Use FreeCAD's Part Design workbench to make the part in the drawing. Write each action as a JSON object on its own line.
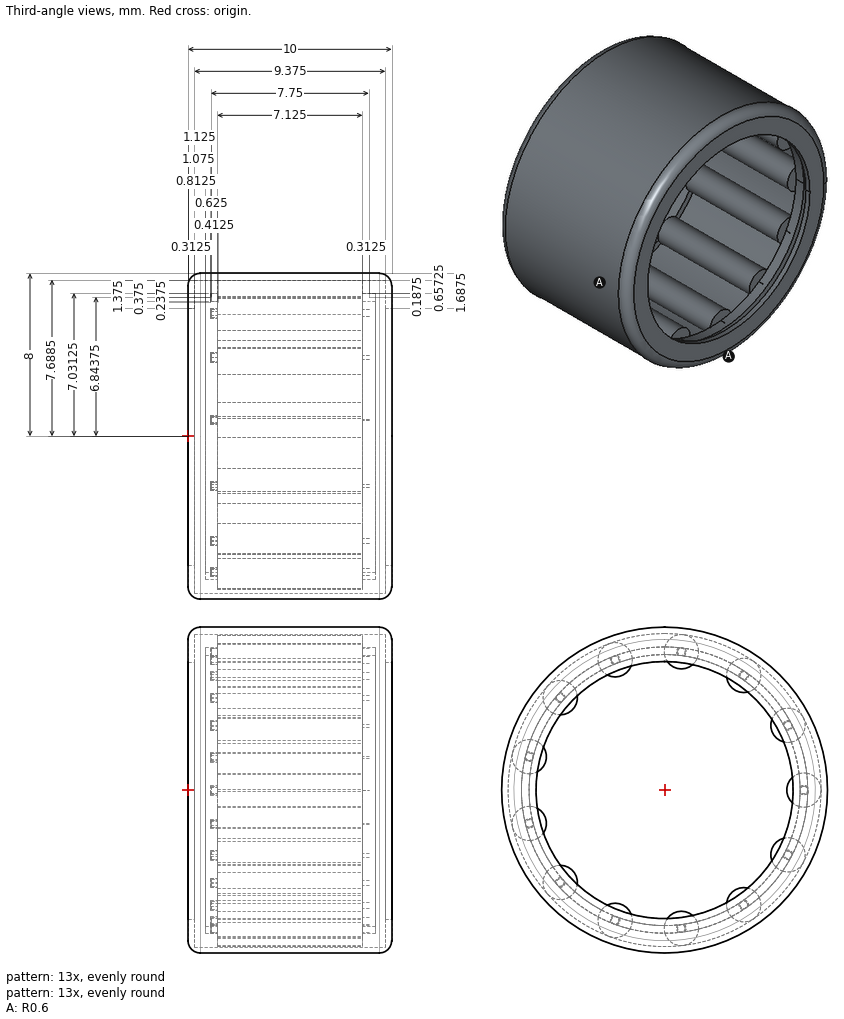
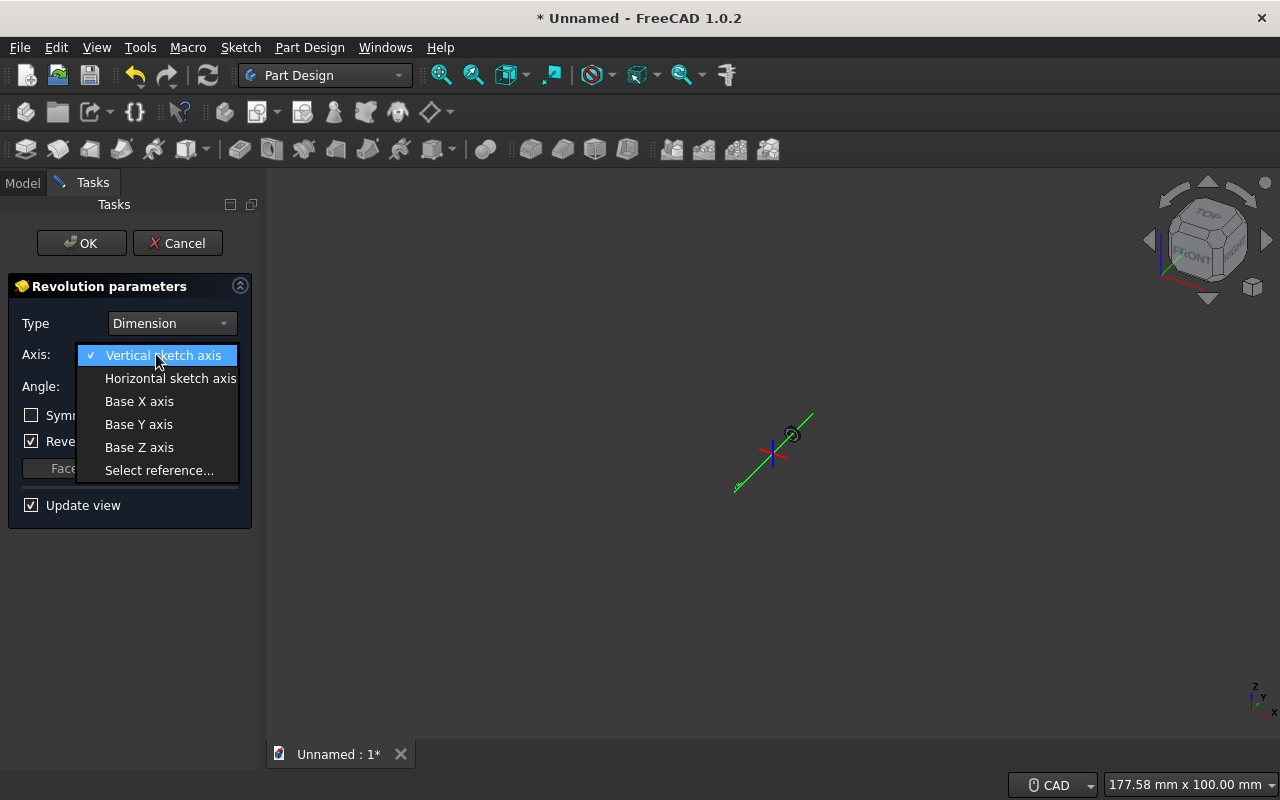
{"action": "left_click", "coordinate": [156, 378]}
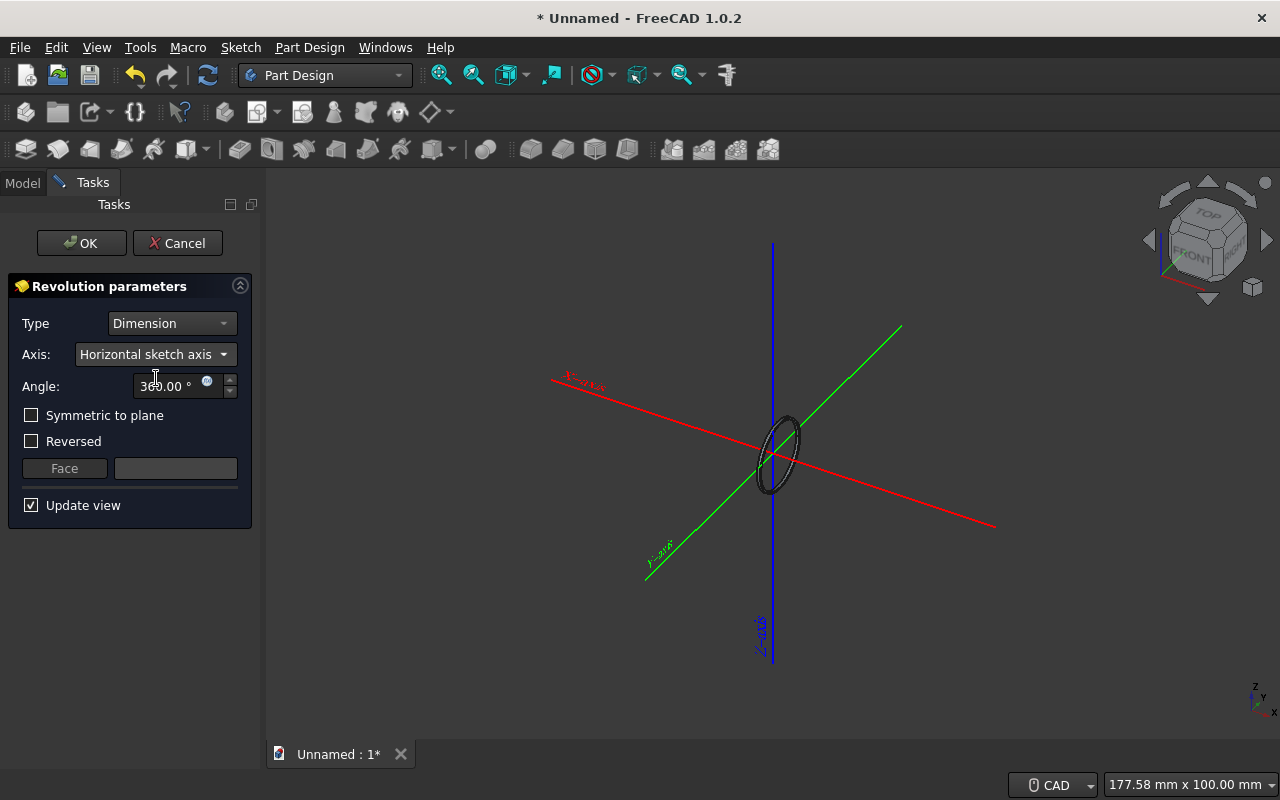
{"action": "left_click", "coordinate": [82, 243]}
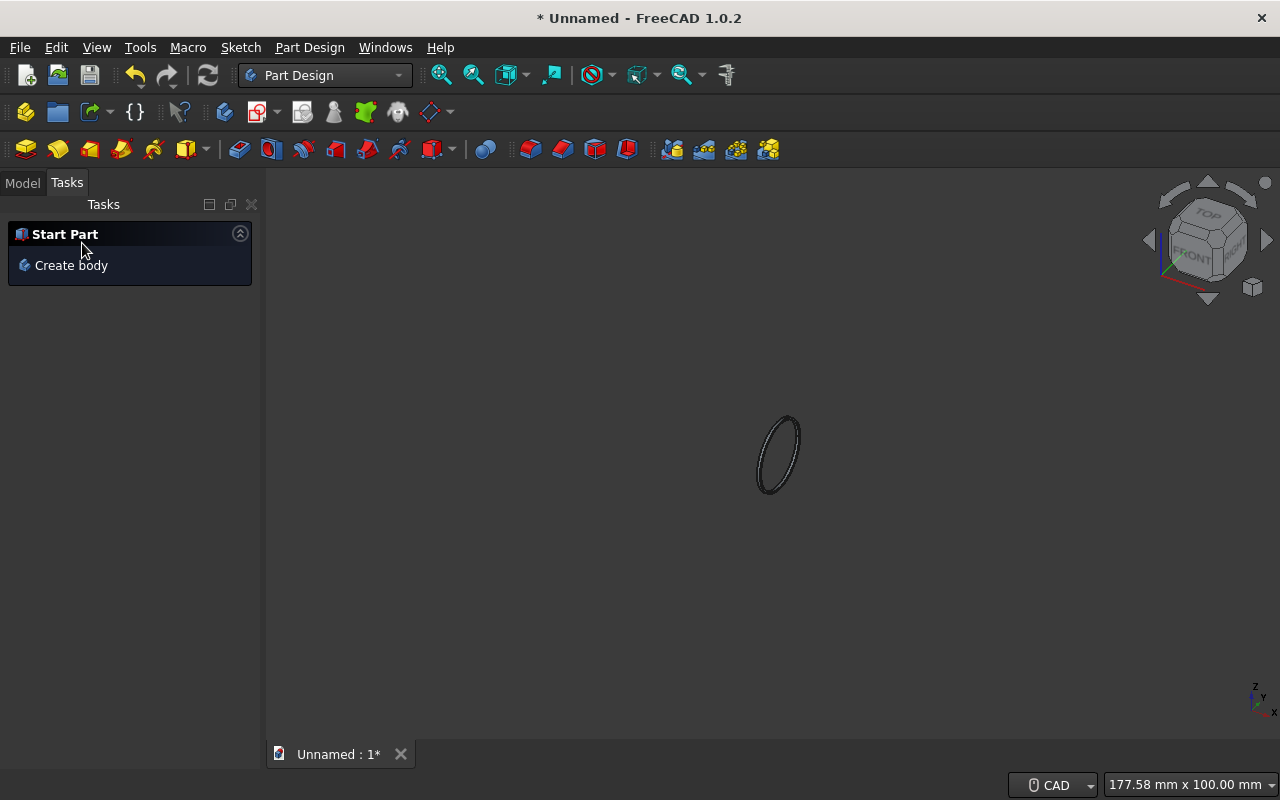
{"action": "left_click", "coordinate": [442, 76]}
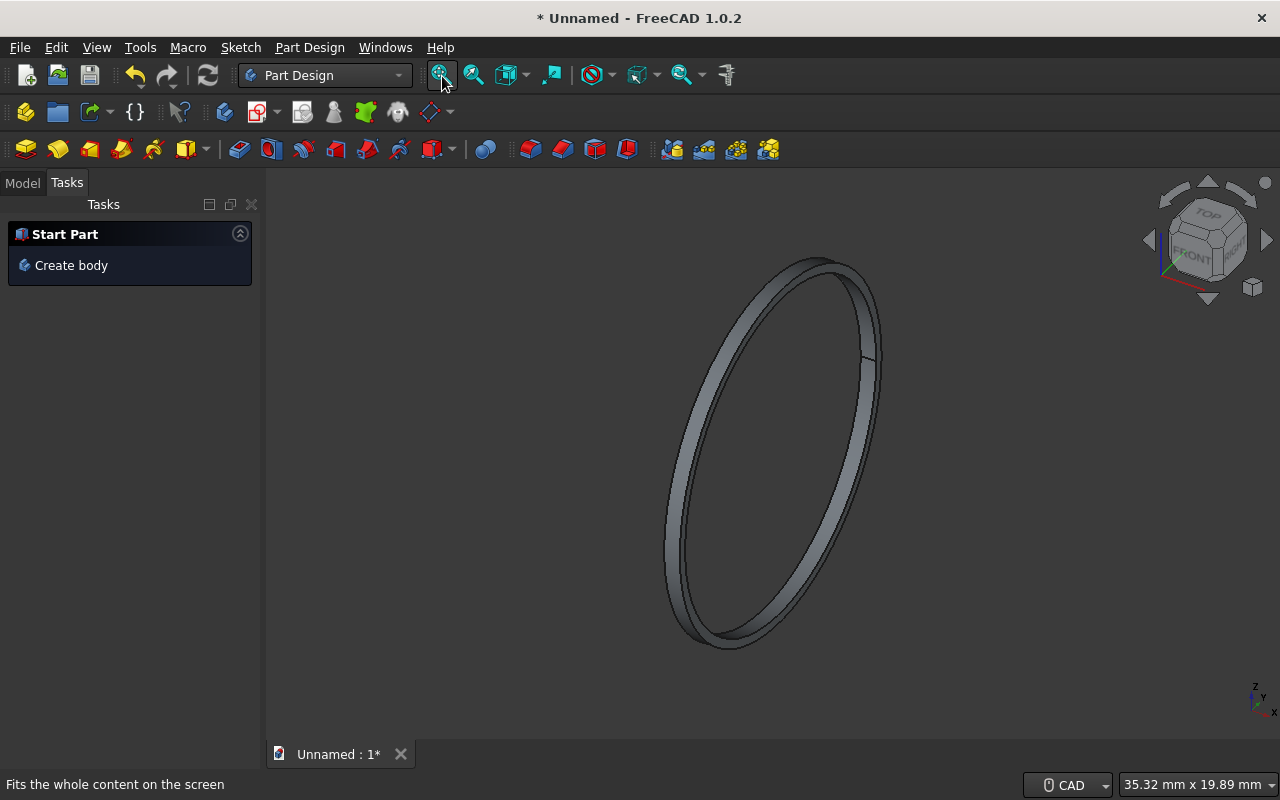
{"action": "left_click", "coordinate": [258, 112]}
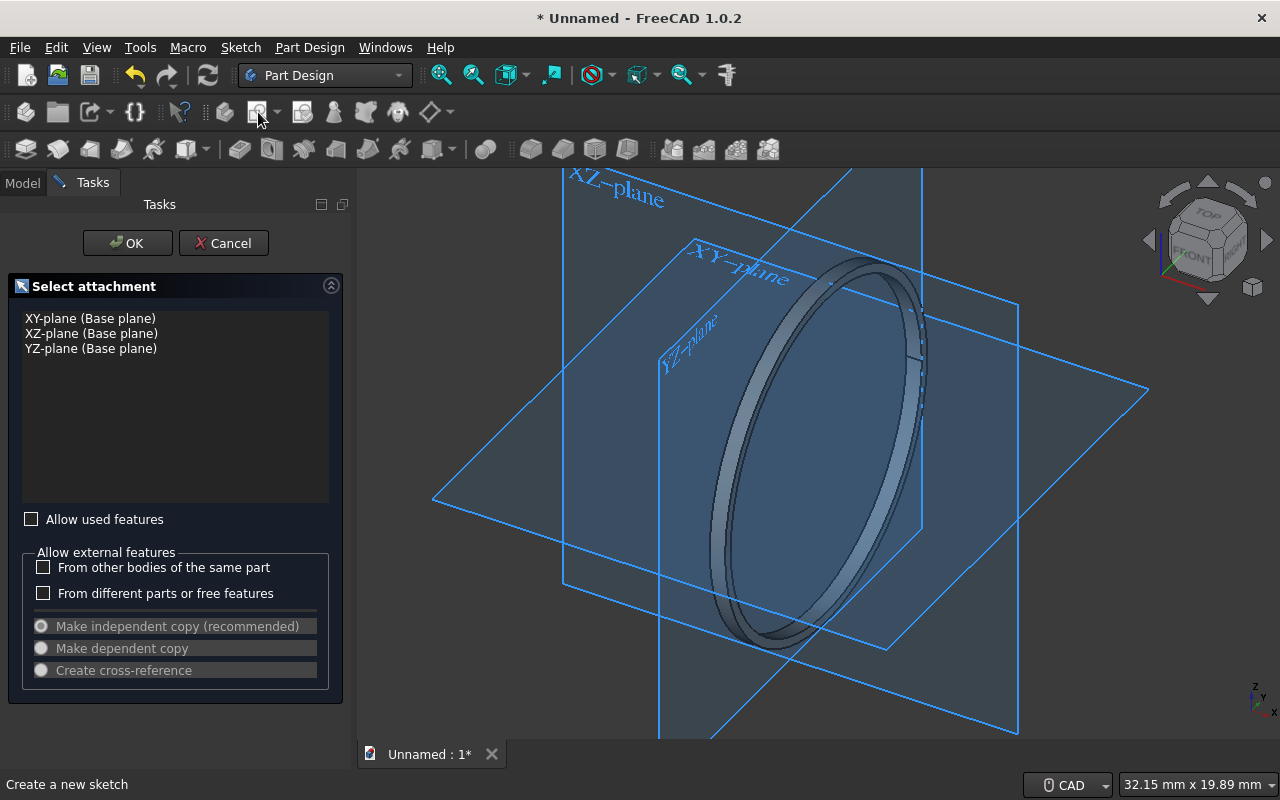
{"action": "left_click", "coordinate": [82, 318]}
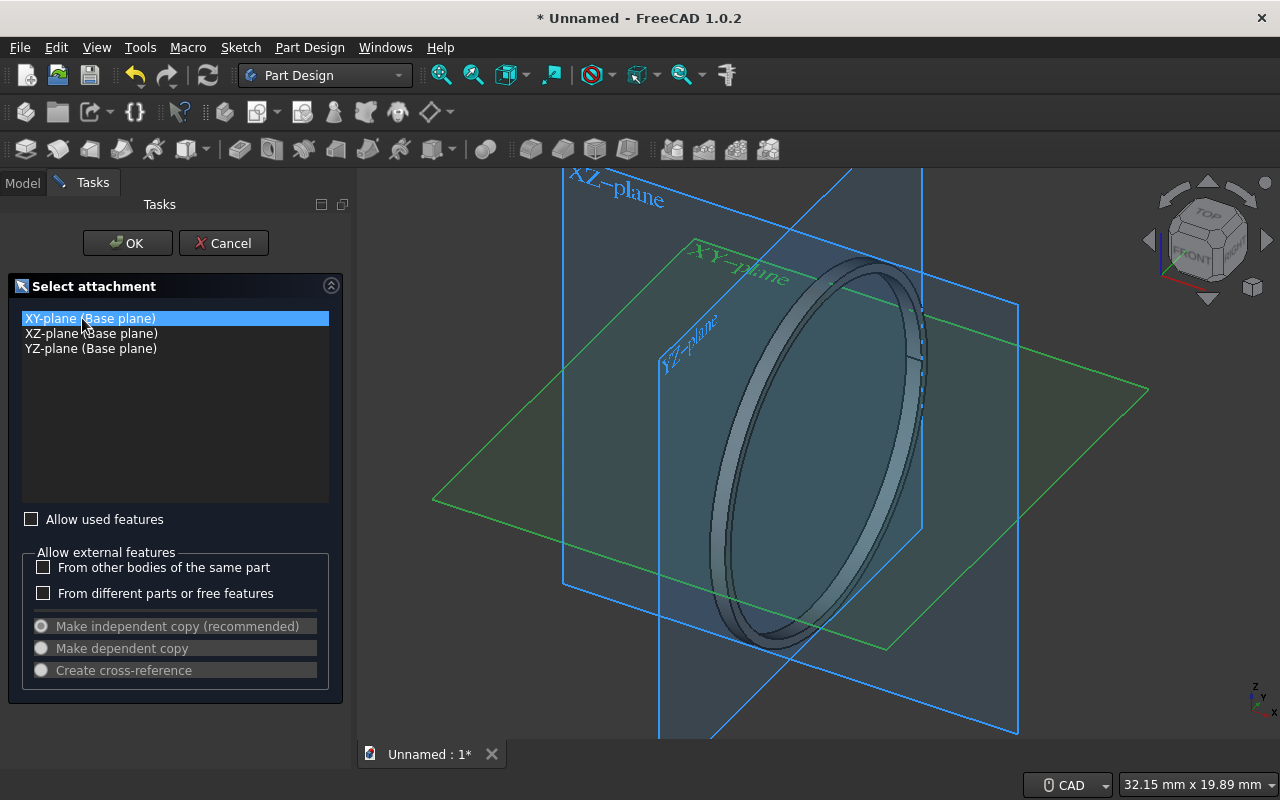
{"action": "left_click", "coordinate": [128, 243]}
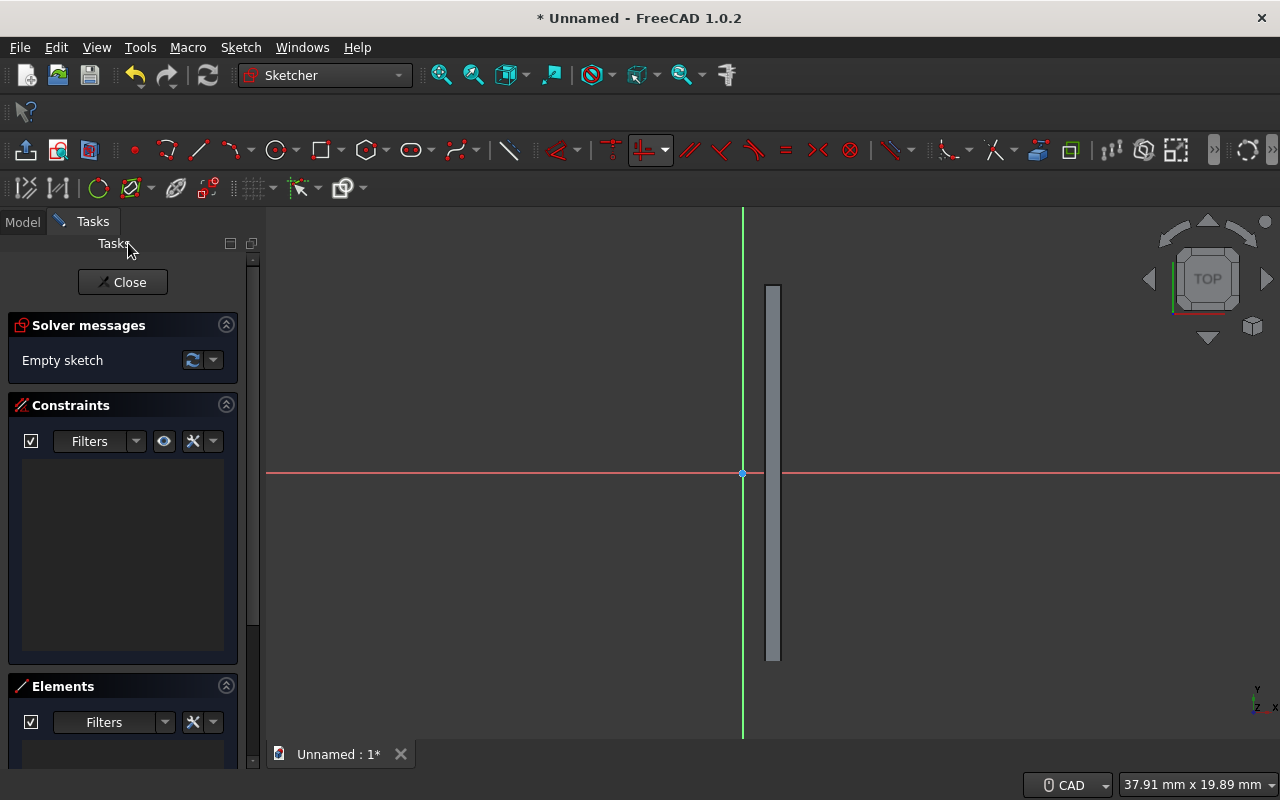
{"action": "left_click", "coordinate": [90, 150]}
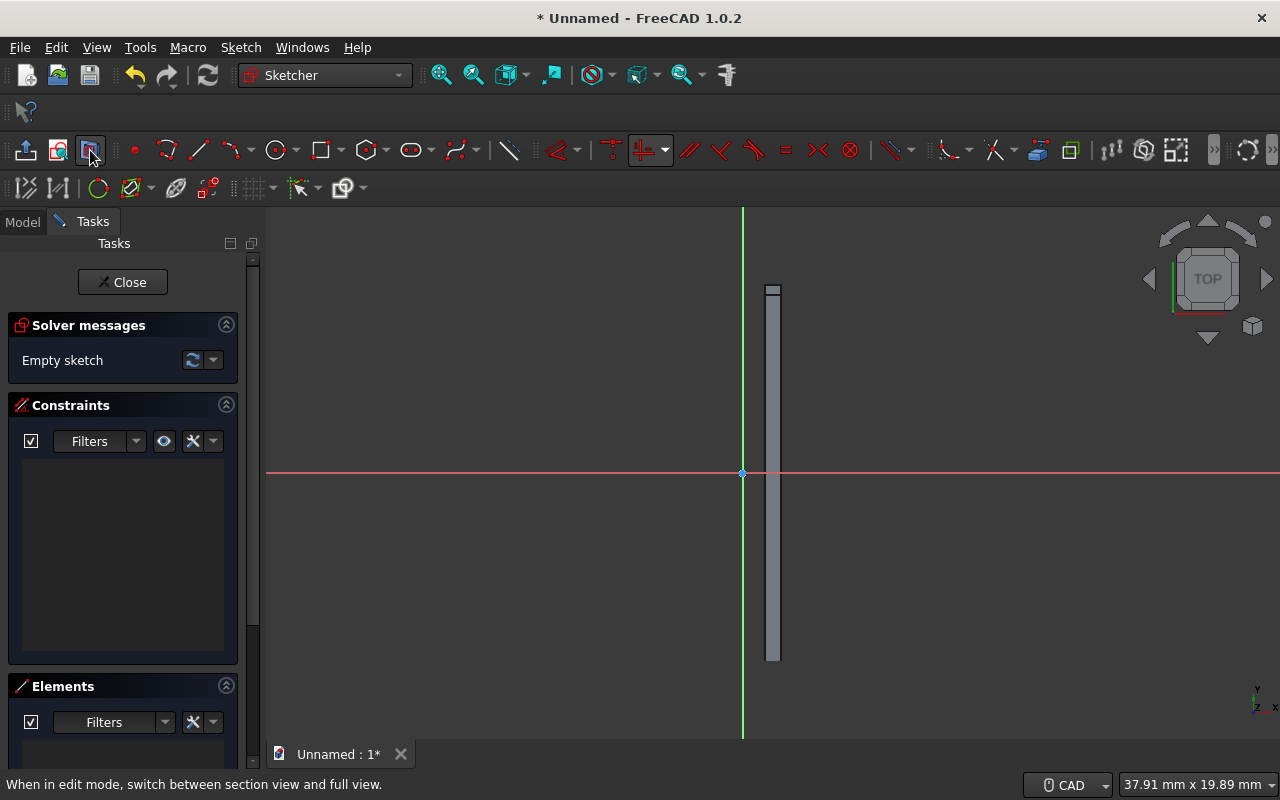
{"action": "scroll", "coordinate": [783, 284], "scroll_direction": "up", "scroll_amount": 15}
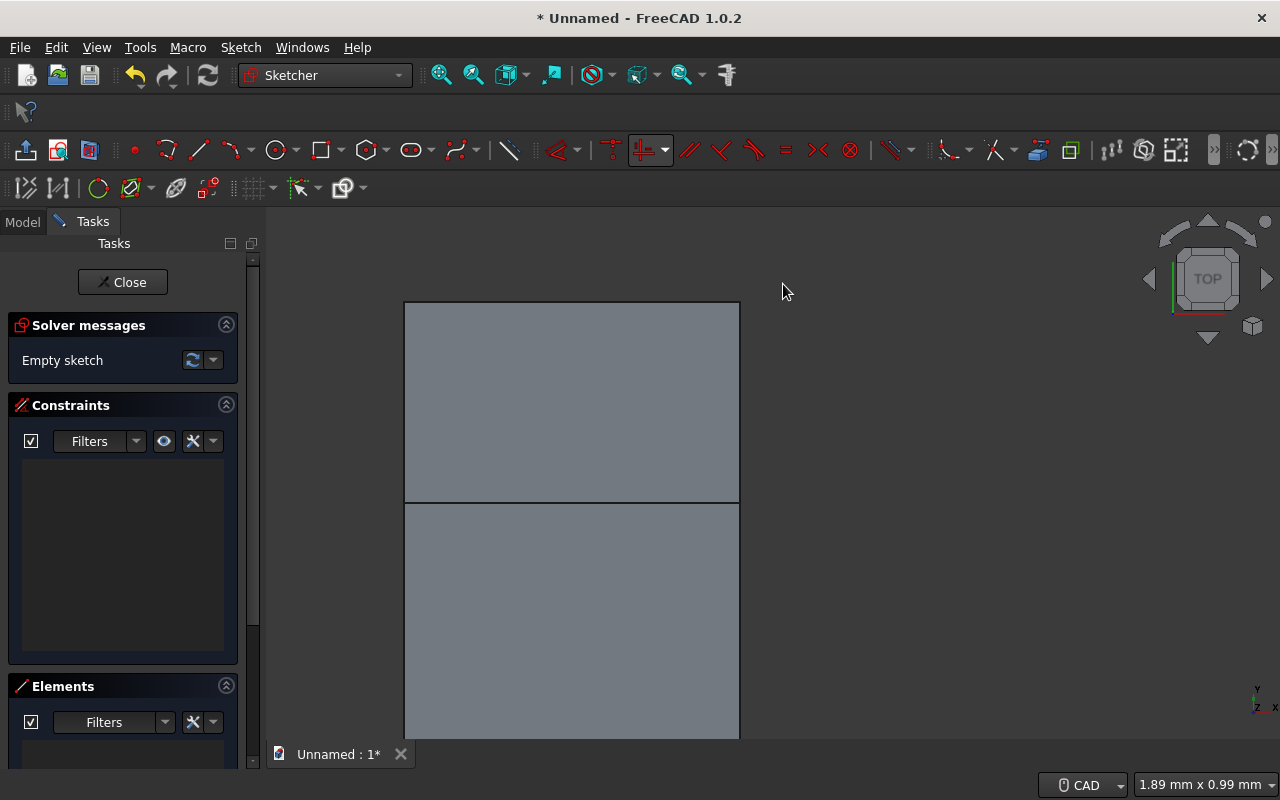
{"action": "scroll", "coordinate": [696, 459], "scroll_direction": "up", "scroll_amount": 3}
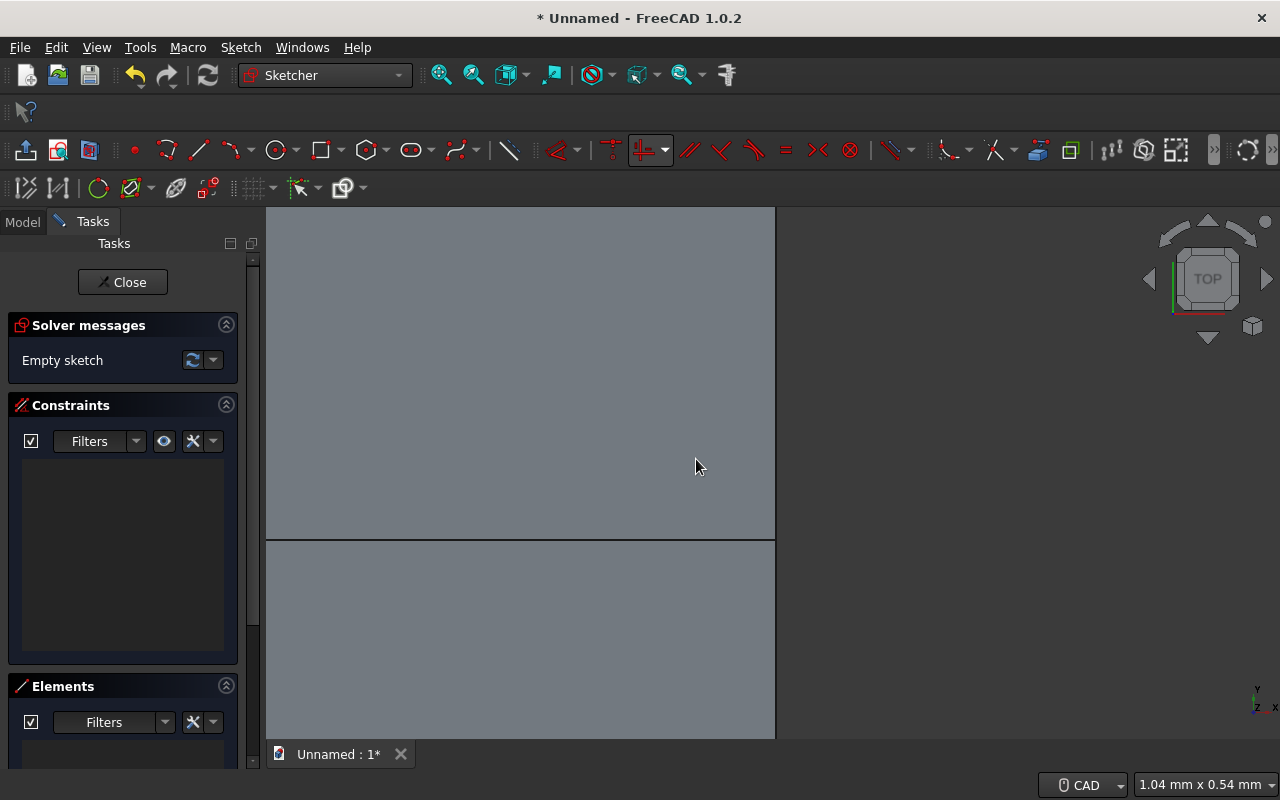
{"action": "left_click", "coordinate": [322, 150]}